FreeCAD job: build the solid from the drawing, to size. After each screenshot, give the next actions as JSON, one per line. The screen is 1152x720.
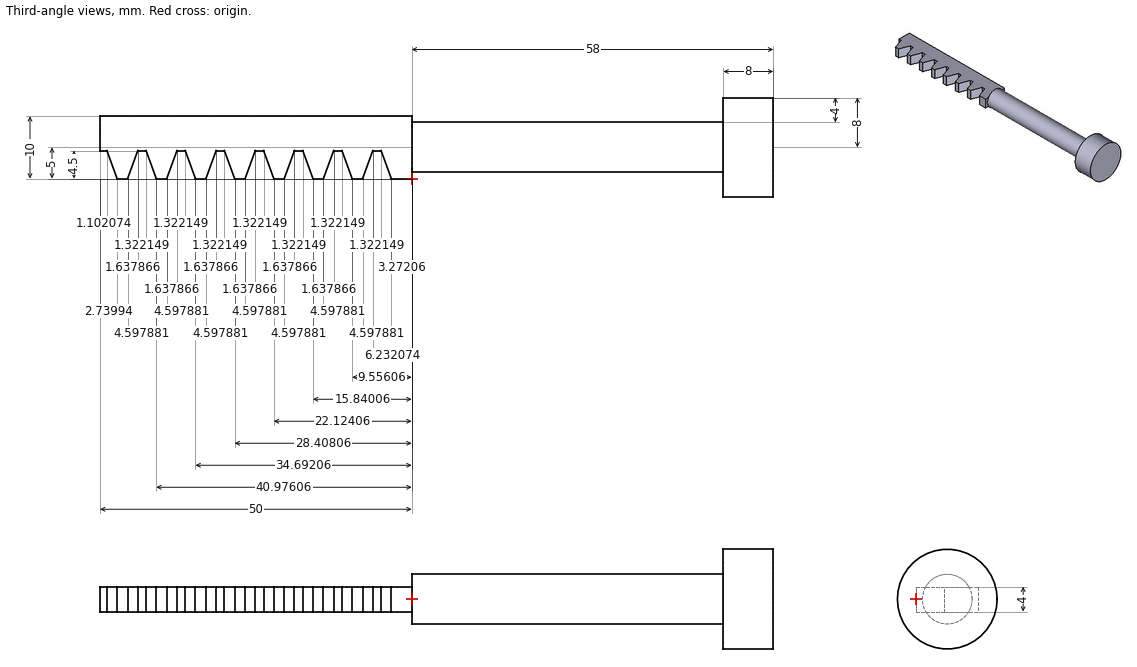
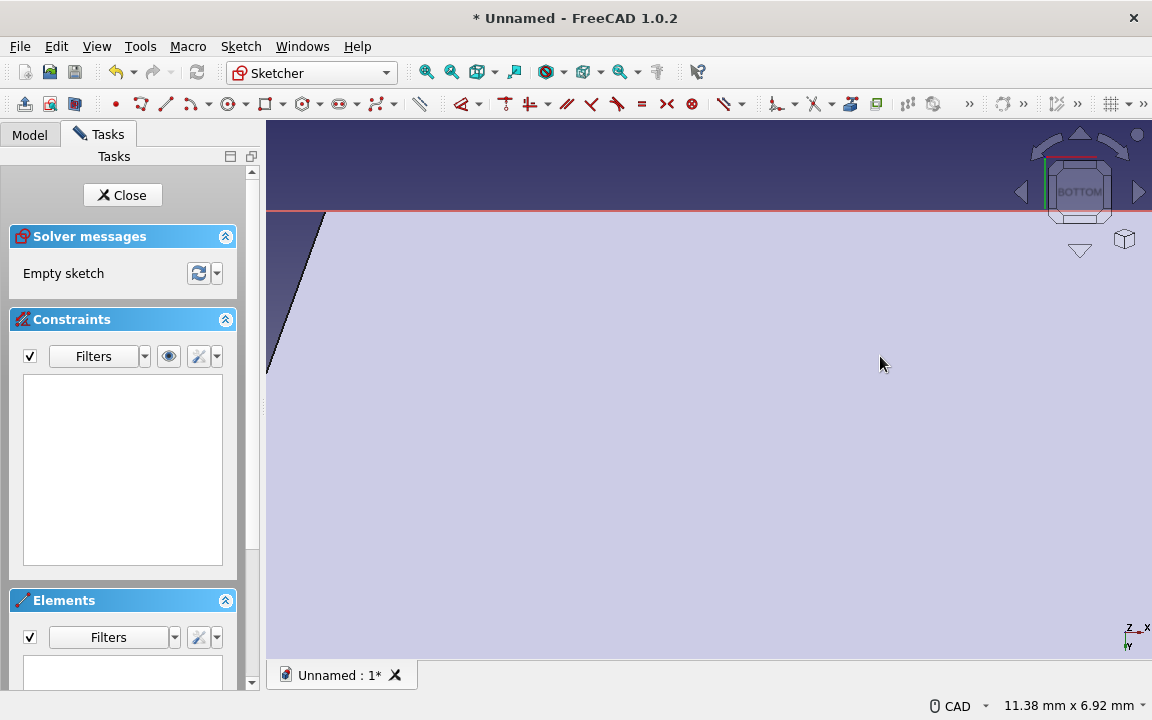
{"action": "left_click", "coordinate": [141, 104]}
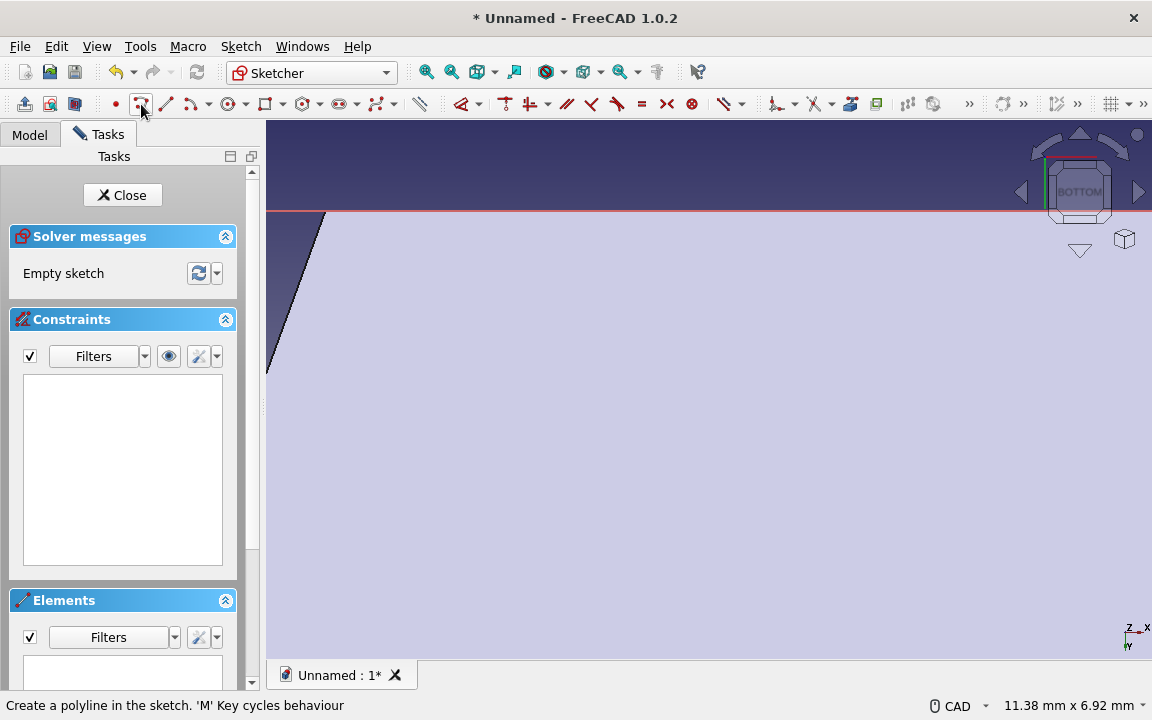
{"action": "left_click", "coordinate": [815, 211]}
{"action": "left_click", "coordinate": [457, 220]}
{"action": "left_click", "coordinate": [584, 562]}
{"action": "left_click", "coordinate": [687, 562]}
{"action": "left_click", "coordinate": [815, 211]}
{"action": "key", "text": "Escape"}
{"action": "key", "text": "Escape"}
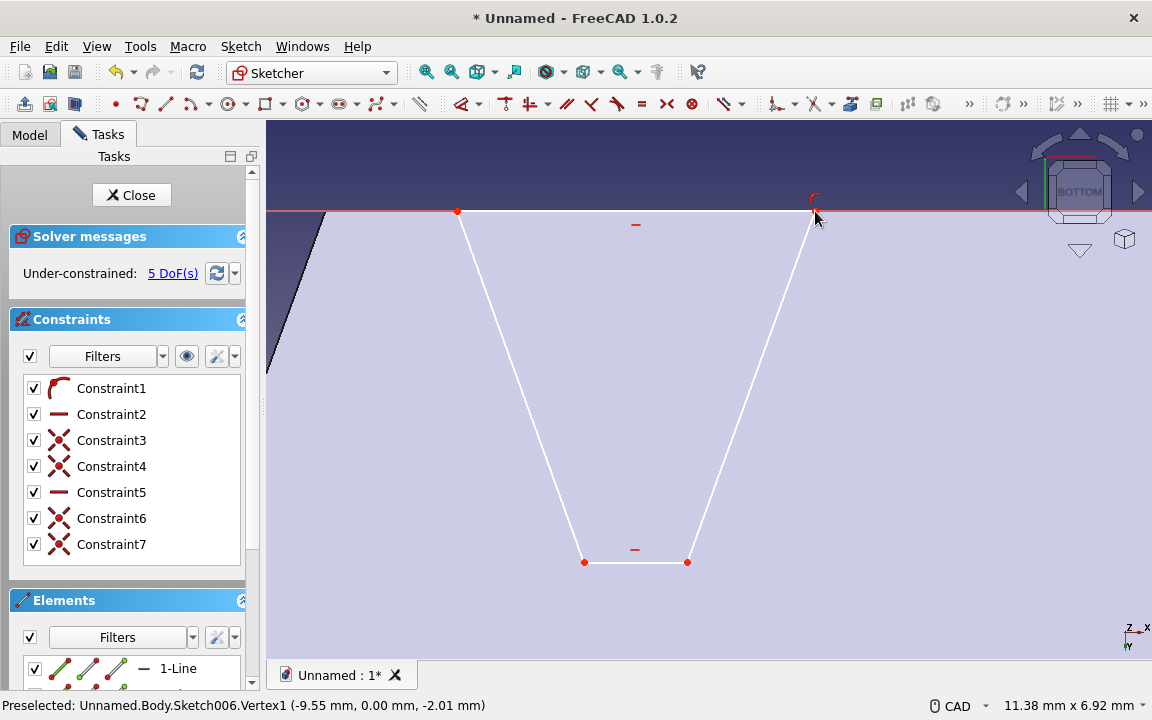
{"action": "left_click", "coordinate": [460, 104]}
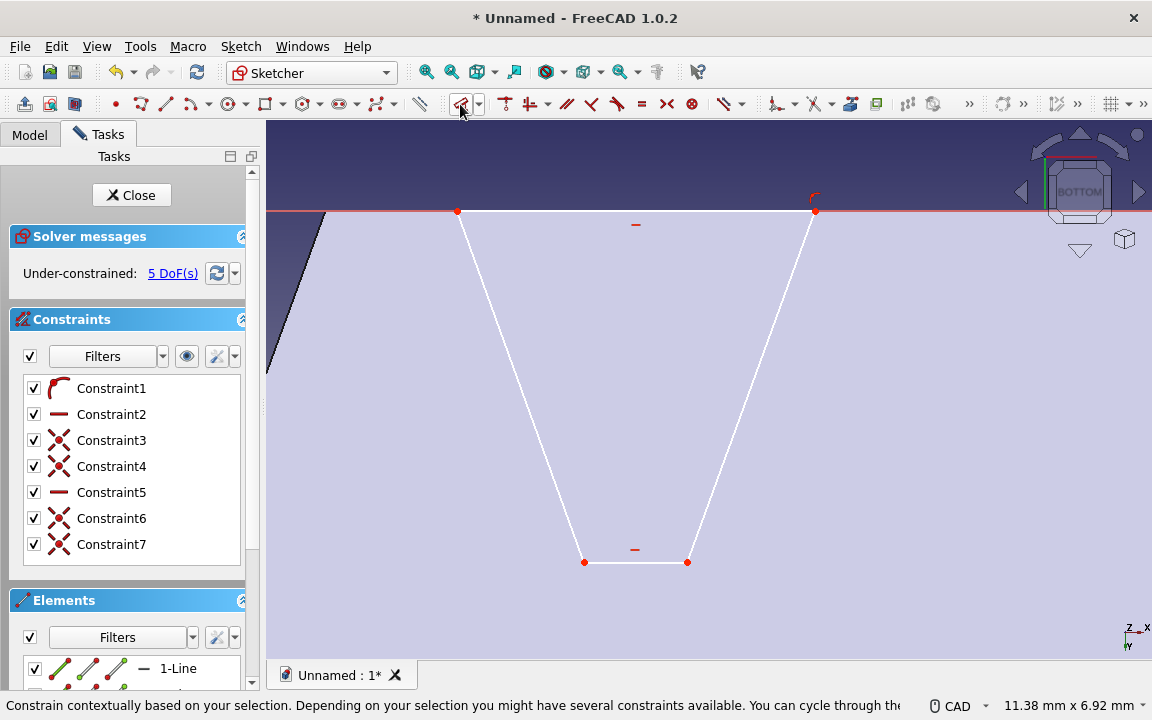
{"action": "left_click", "coordinate": [584, 563]}
{"action": "left_click", "coordinate": [550, 387]}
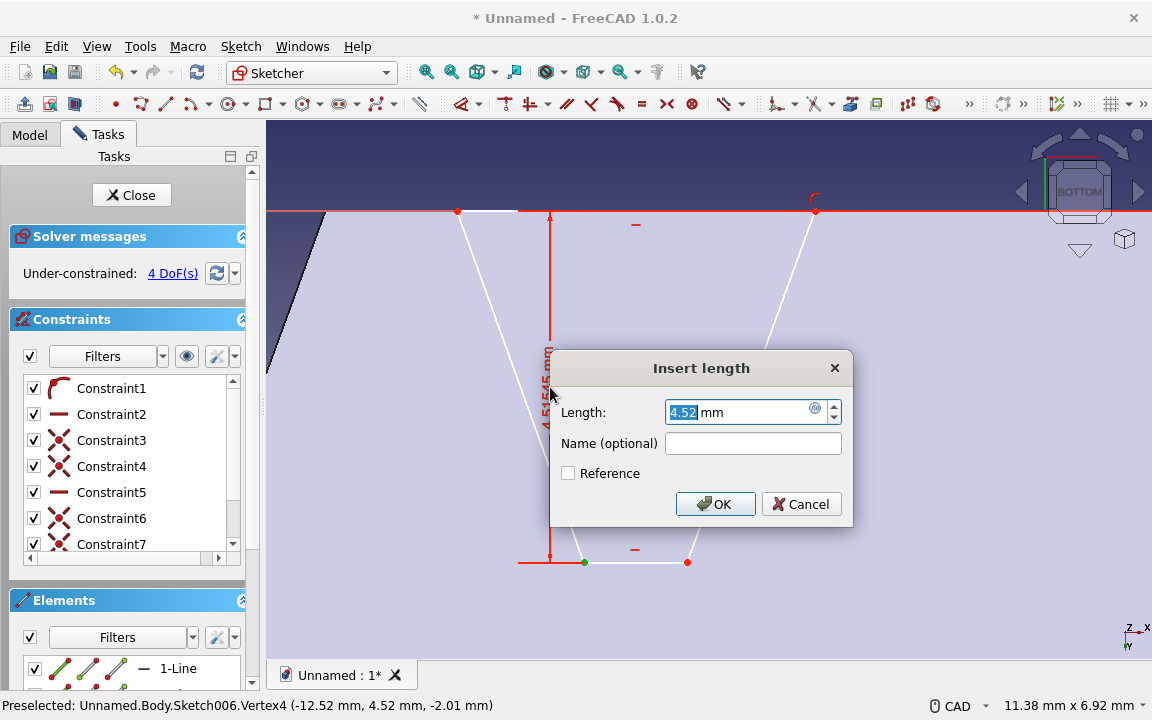
{"action": "type", "text": "4.5"}
{"action": "key", "text": "Return"}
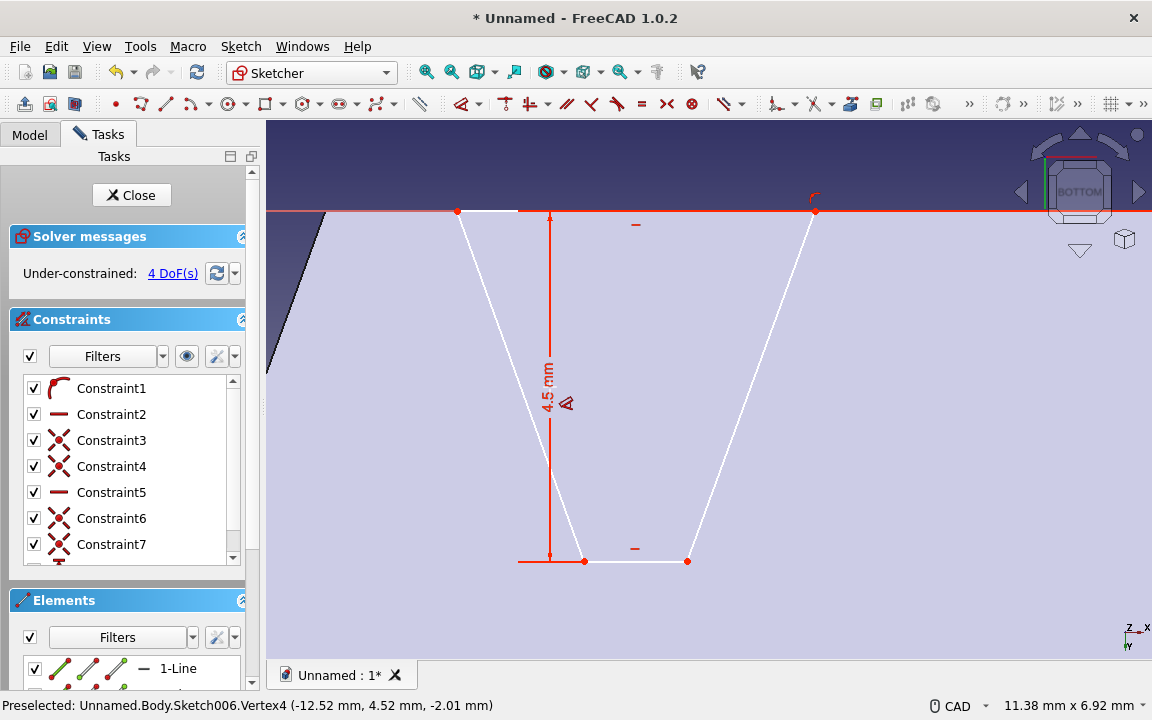
{"action": "left_click", "coordinate": [708, 211]}
{"action": "left_click", "coordinate": [636, 177]}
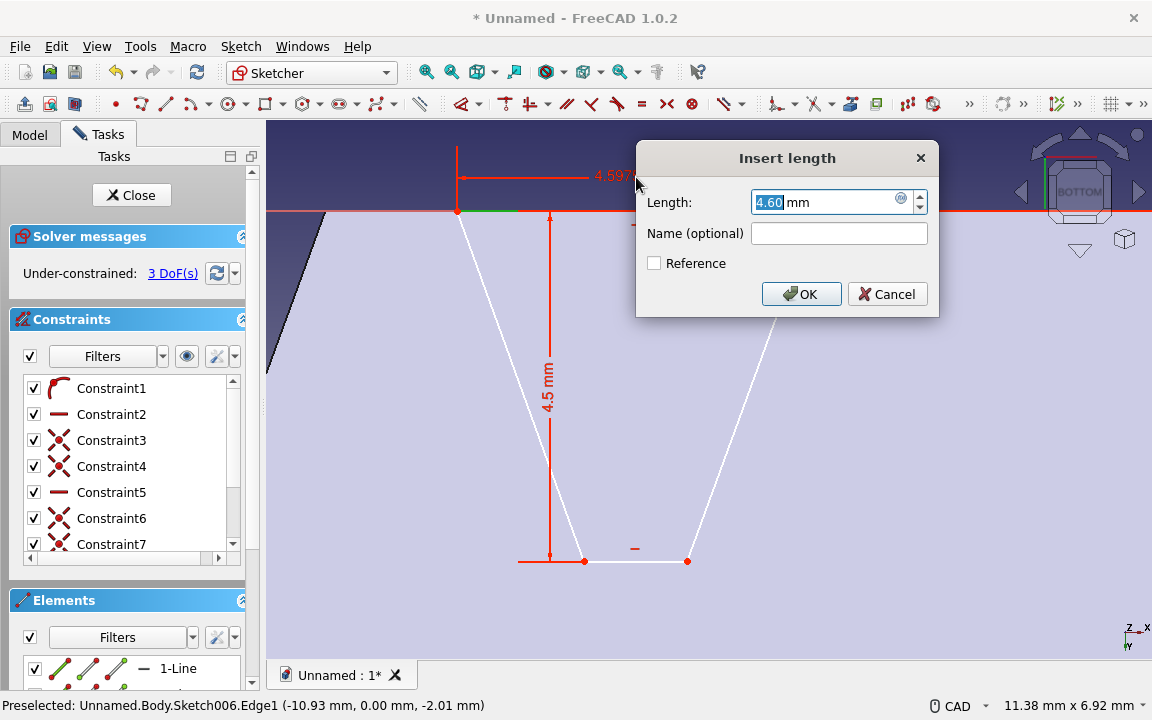
{"action": "type", "text": "4.597881"}
{"action": "key", "text": "Return"}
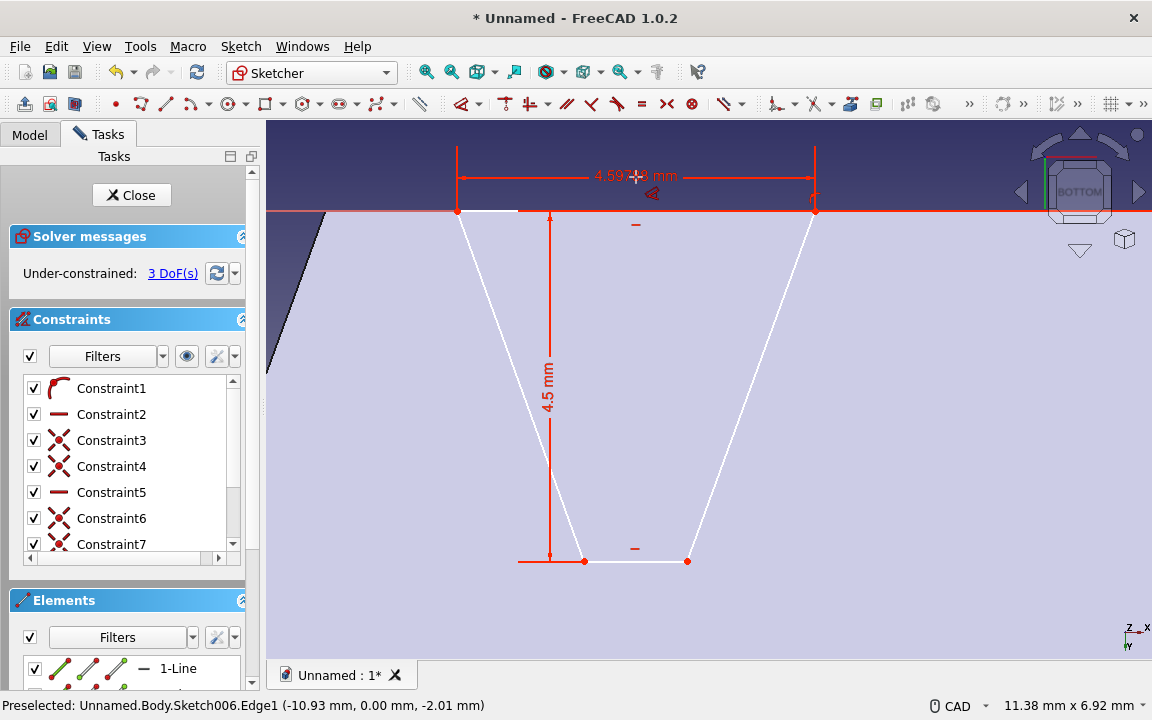
{"action": "left_click", "coordinate": [615, 562]}
{"action": "left_click", "coordinate": [635, 596]}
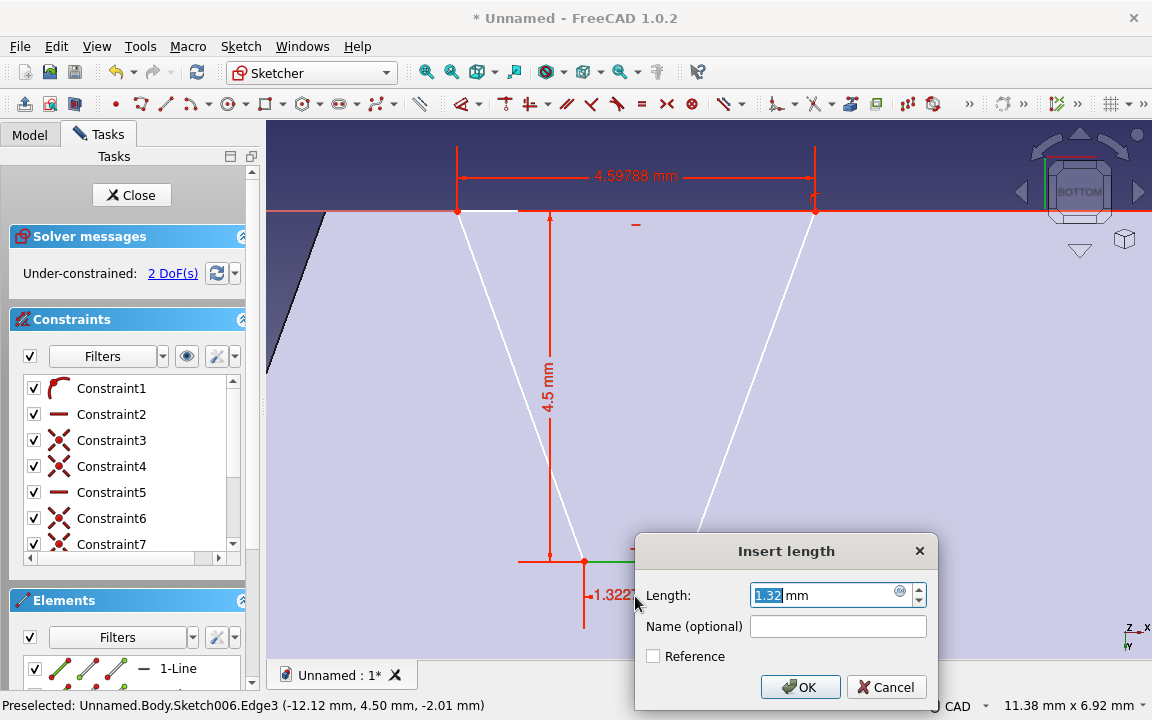
{"action": "type", "text": "1.322149"}
{"action": "key", "text": "Return"}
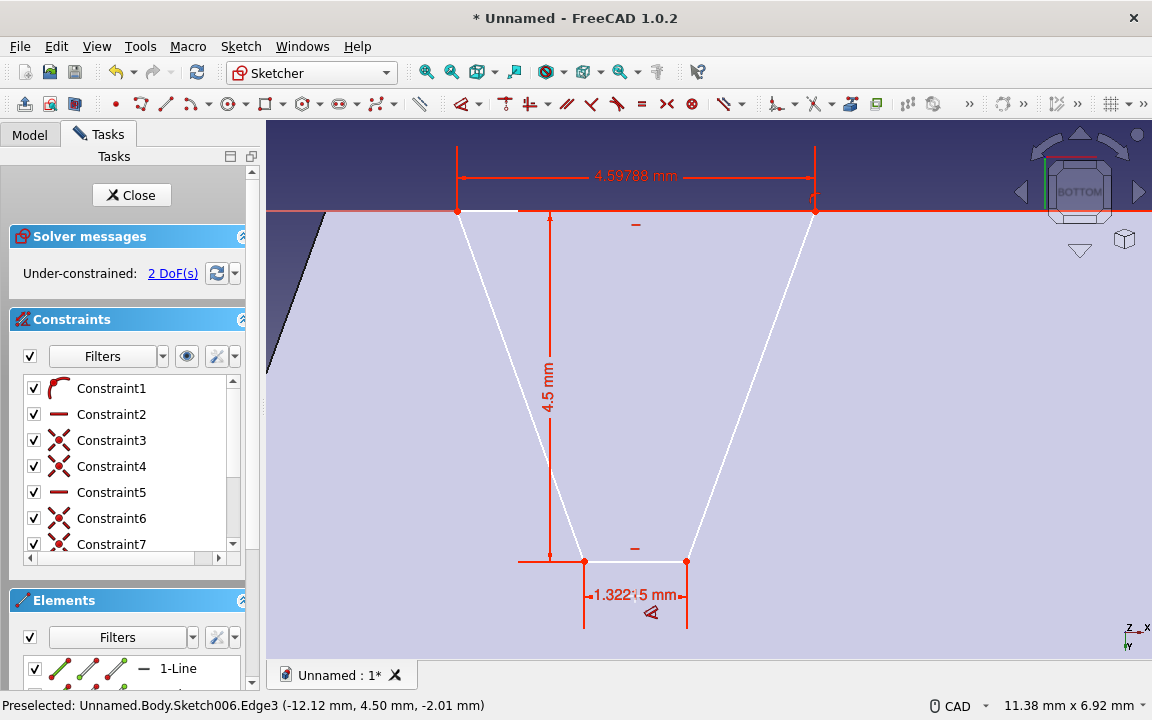
{"action": "left_click", "coordinate": [815, 211]}
{"action": "left_click", "coordinate": [901, 177]}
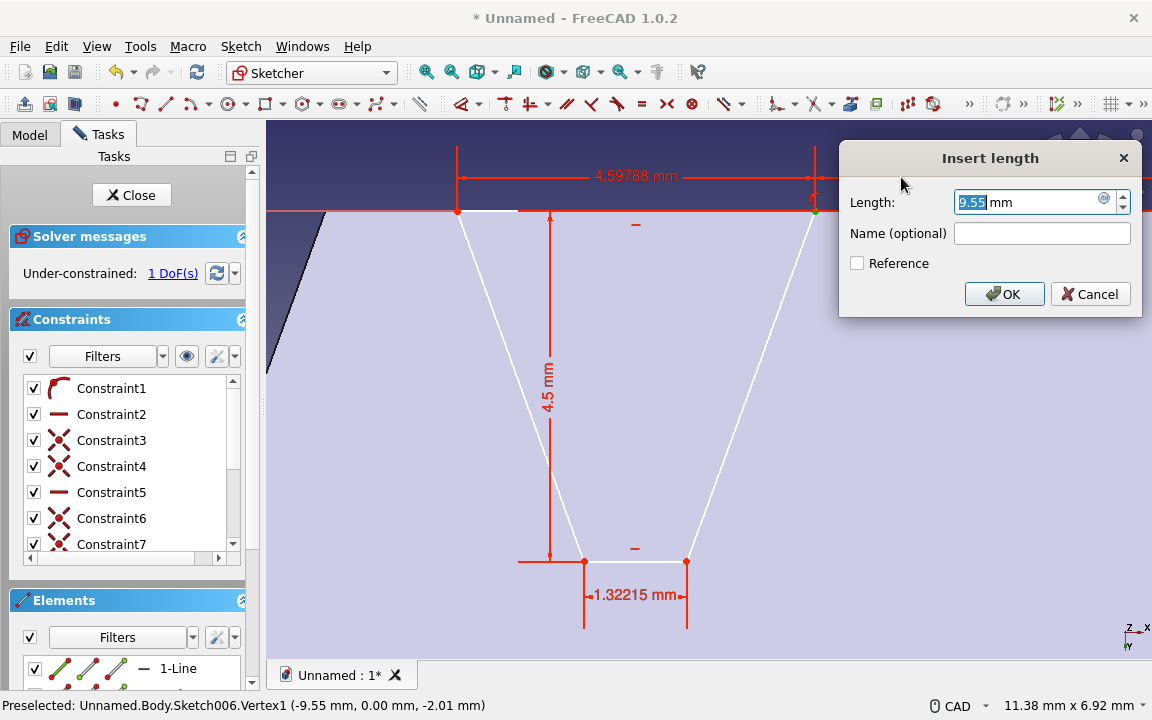
{"action": "type", "text": "9.55606"}
{"action": "key", "text": "Return"}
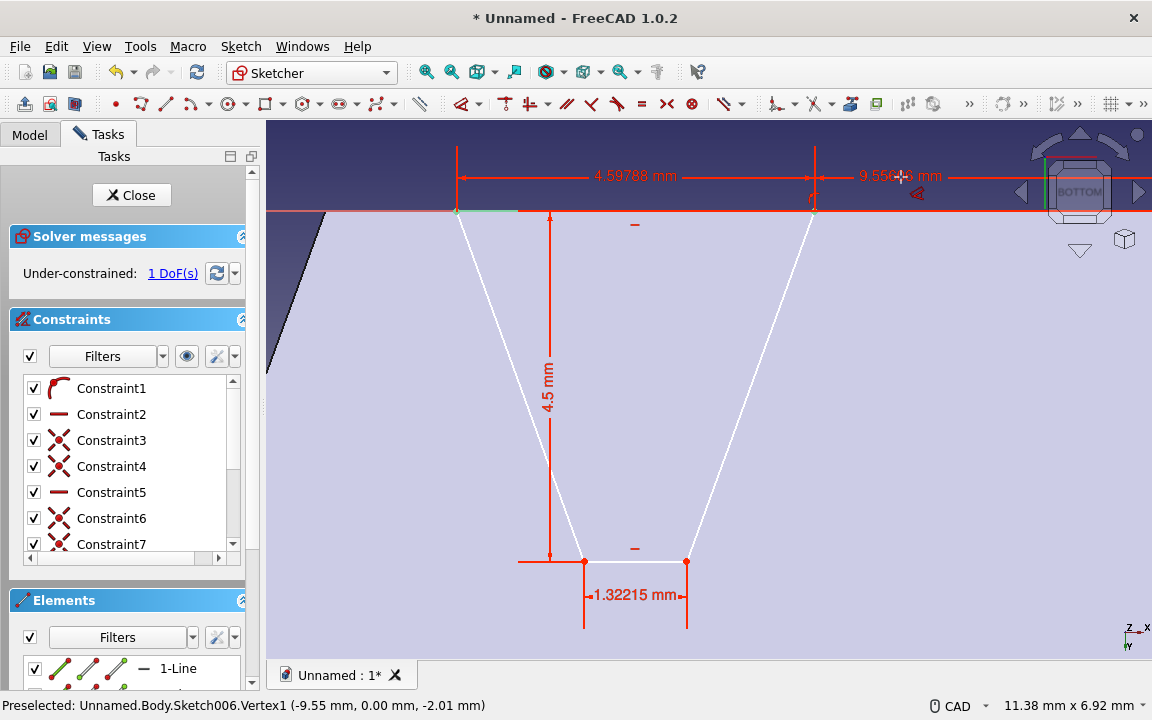
{"action": "left_click", "coordinate": [495, 317]}
{"action": "left_click", "coordinate": [520, 596]}